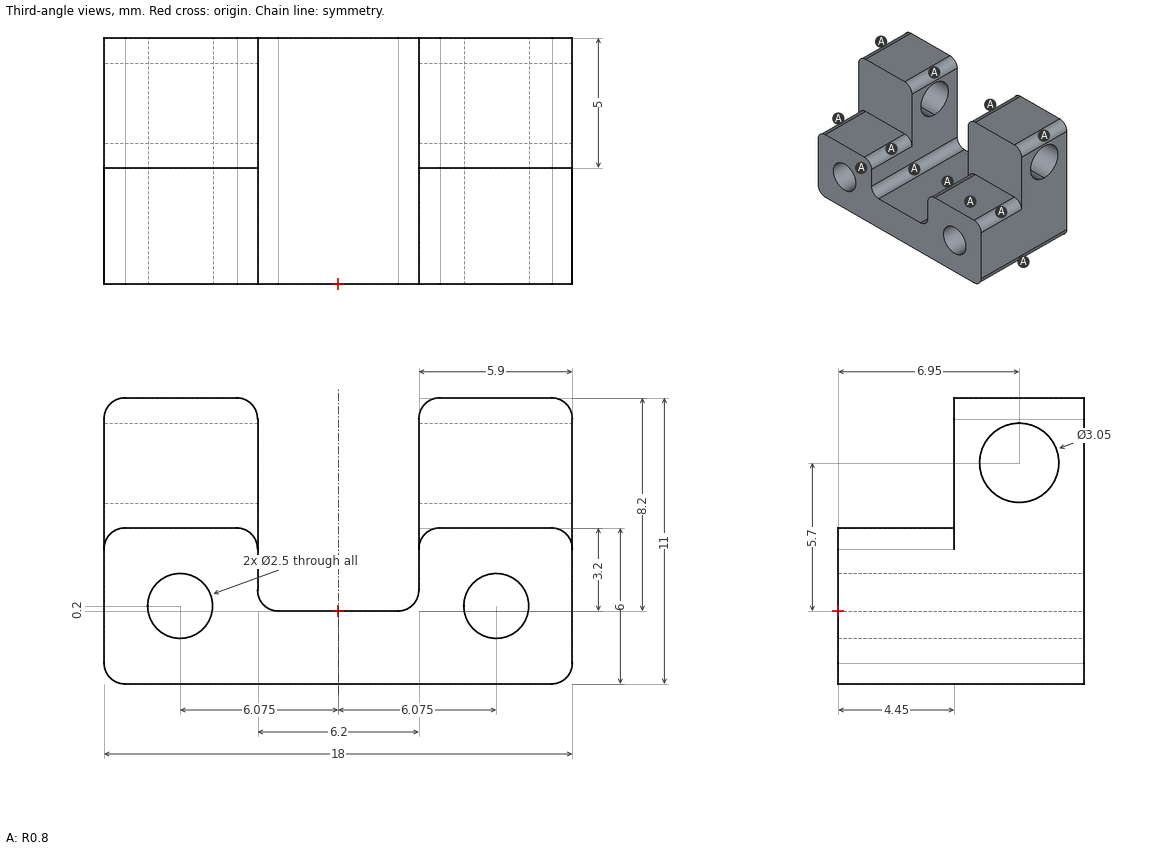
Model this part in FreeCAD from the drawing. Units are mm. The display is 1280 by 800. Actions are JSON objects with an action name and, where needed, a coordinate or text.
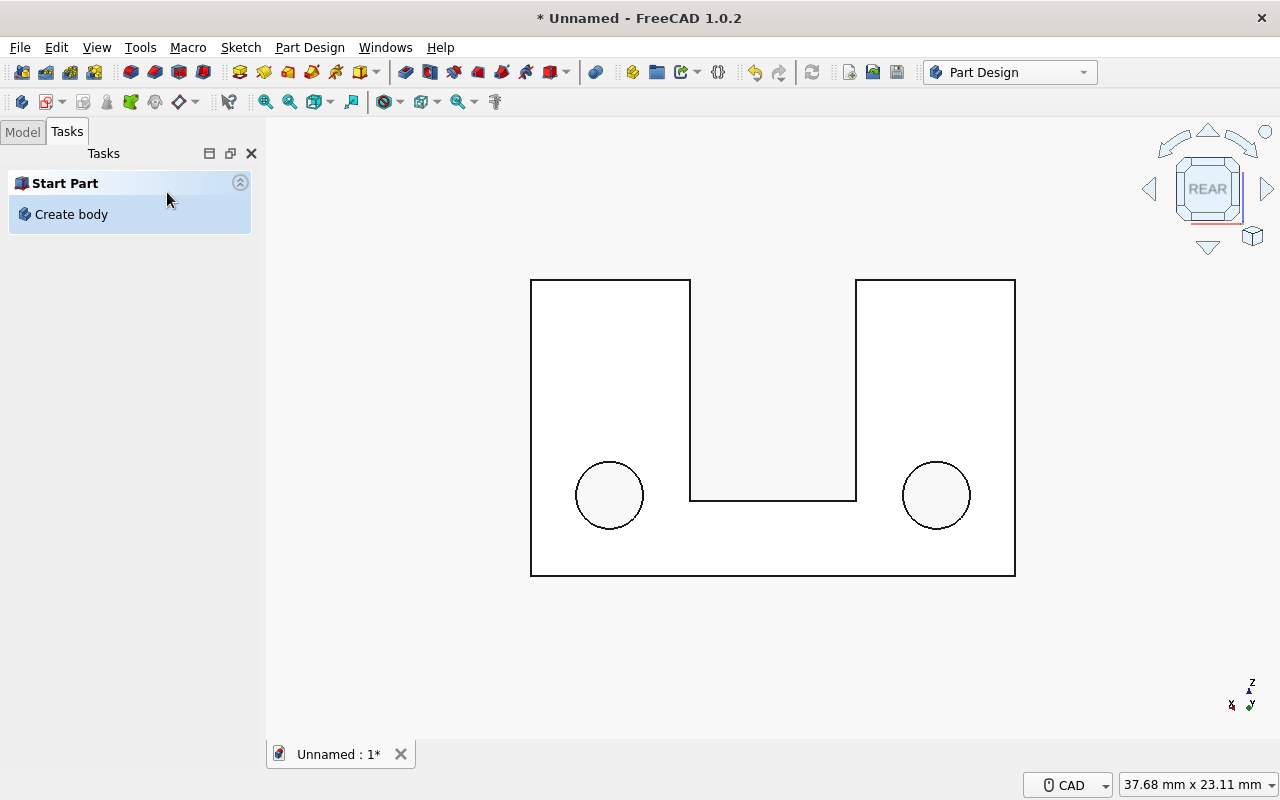
{"action": "key", "text": "6"}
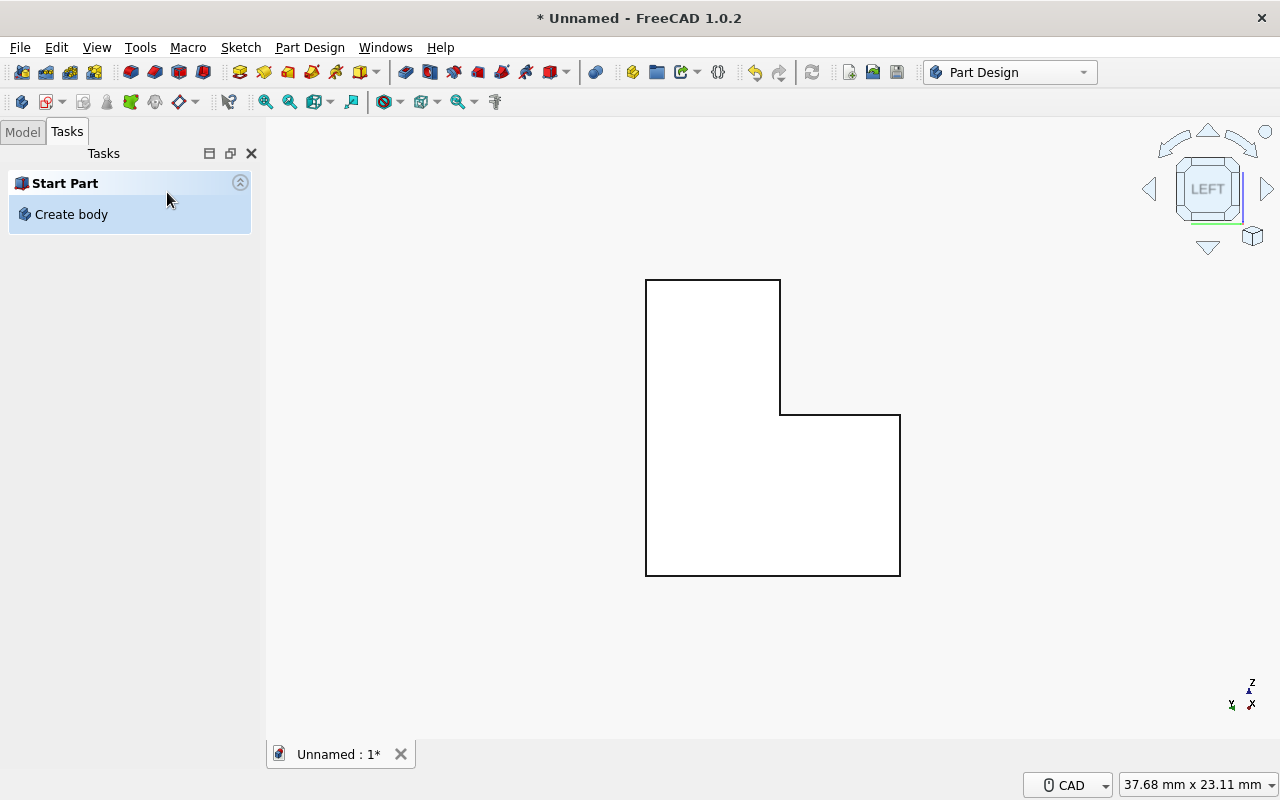
{"action": "left_click", "coordinate": [737, 469]}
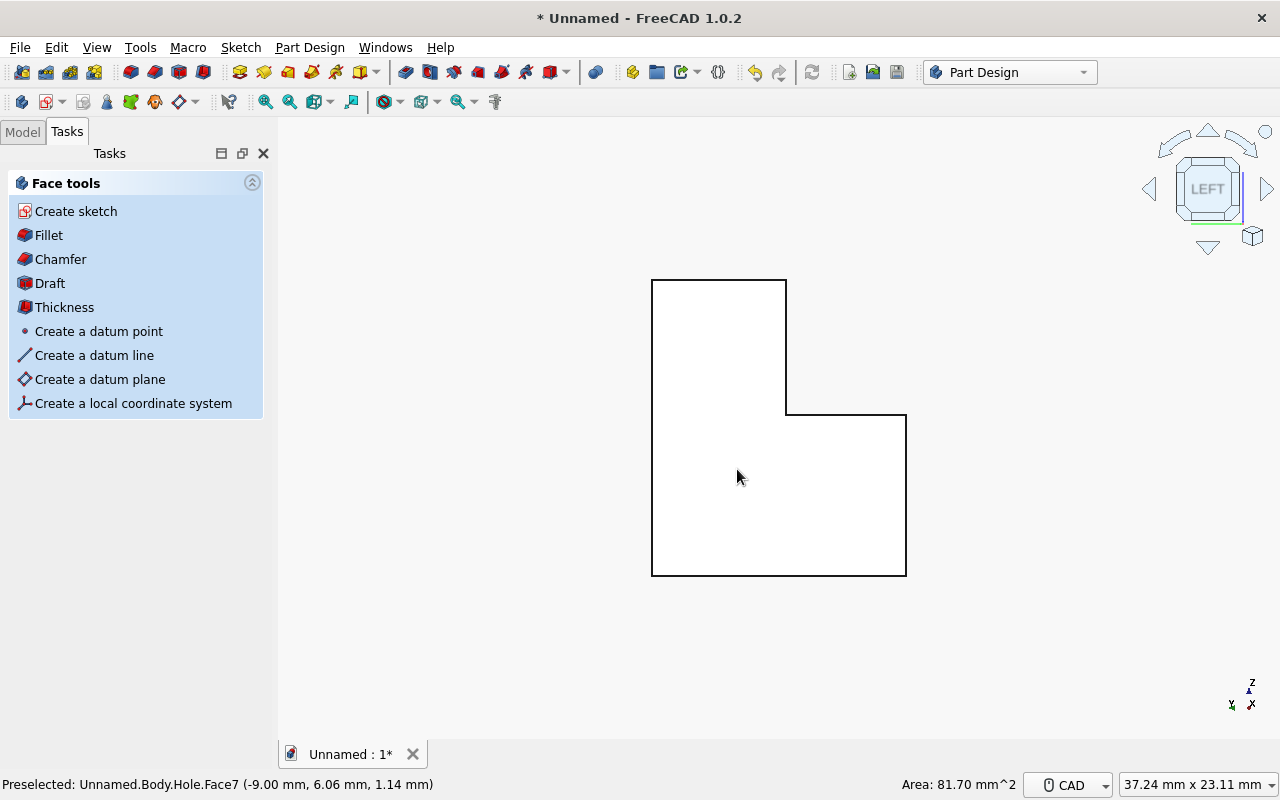
{"action": "left_click", "coordinate": [46, 102]}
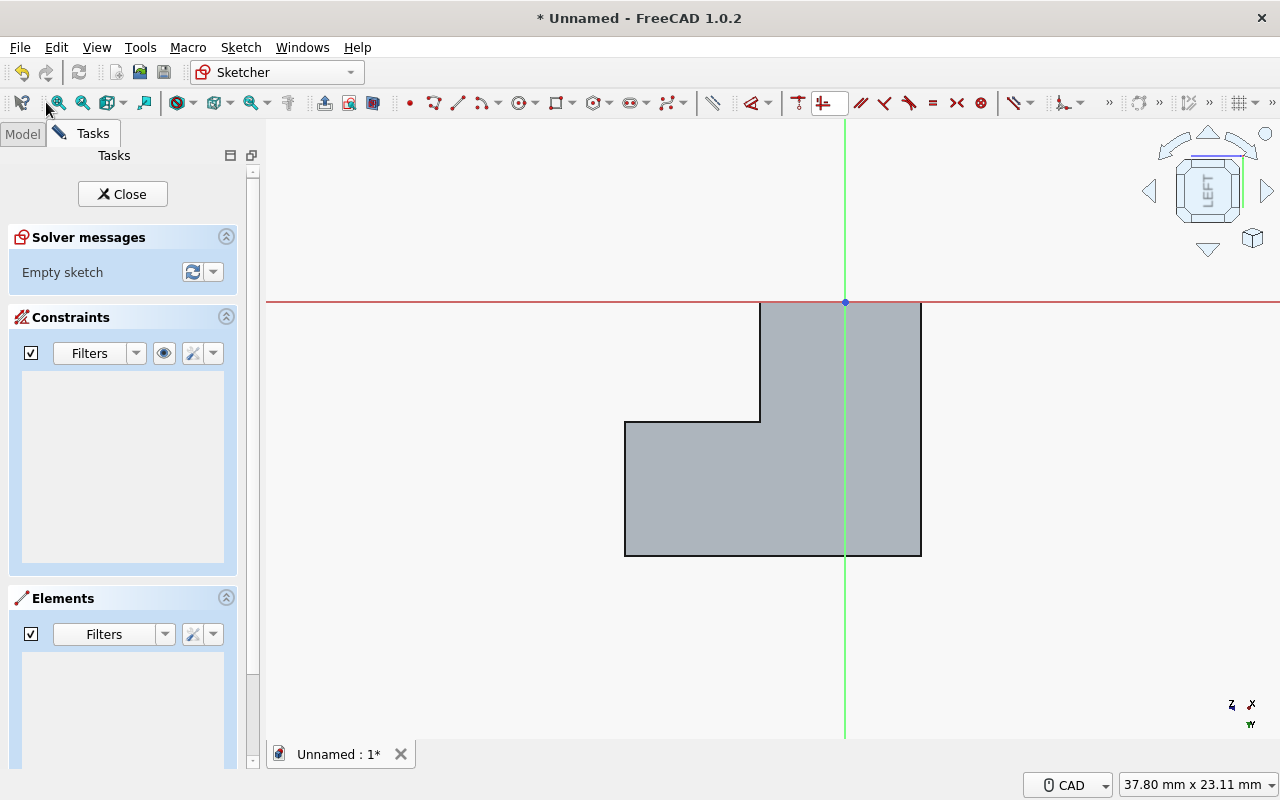
{"action": "scroll", "coordinate": [690, 504], "scroll_direction": "up", "scroll_amount": 8}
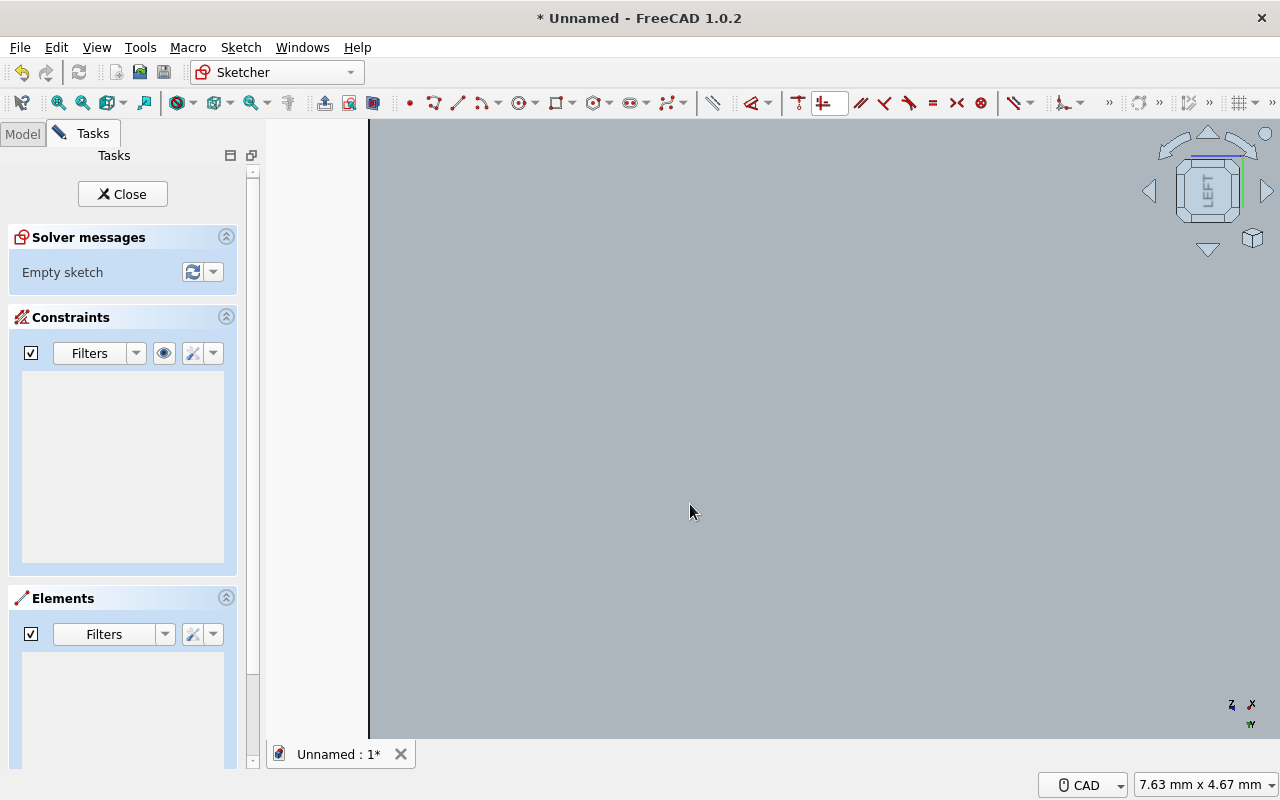
{"action": "left_click", "coordinate": [520, 104]}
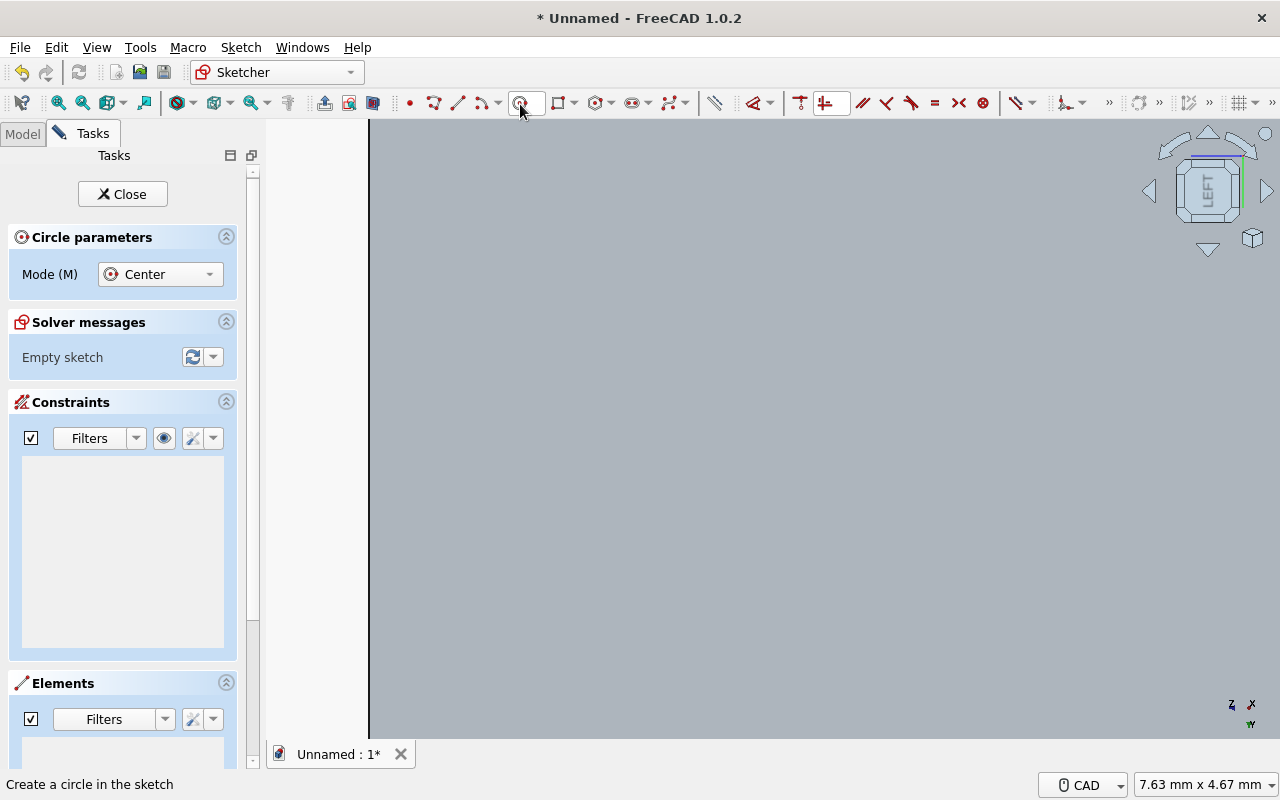
{"action": "left_click", "coordinate": [701, 426]}
{"action": "mouse_move", "coordinate": [844, 282]}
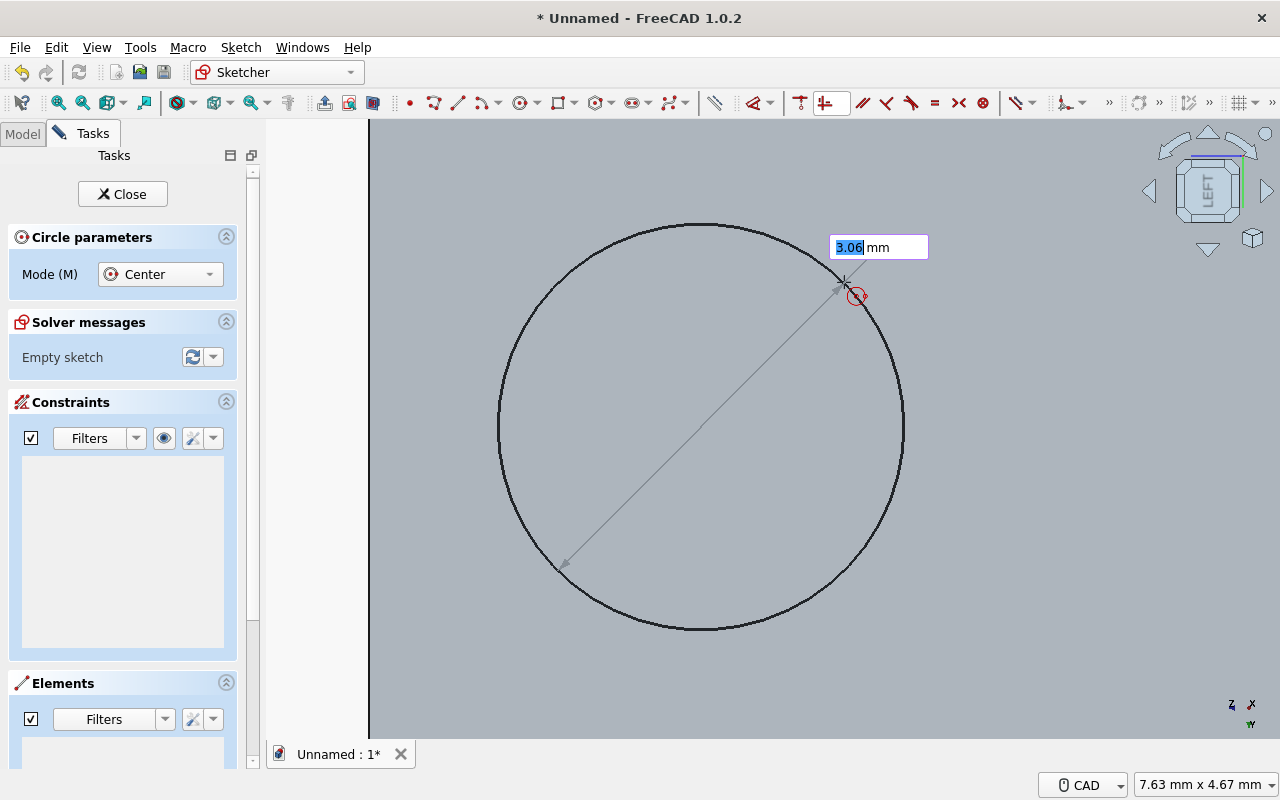
{"action": "type", "text": "3.05"}
{"action": "key", "text": "Return"}
{"action": "key", "text": "Escape"}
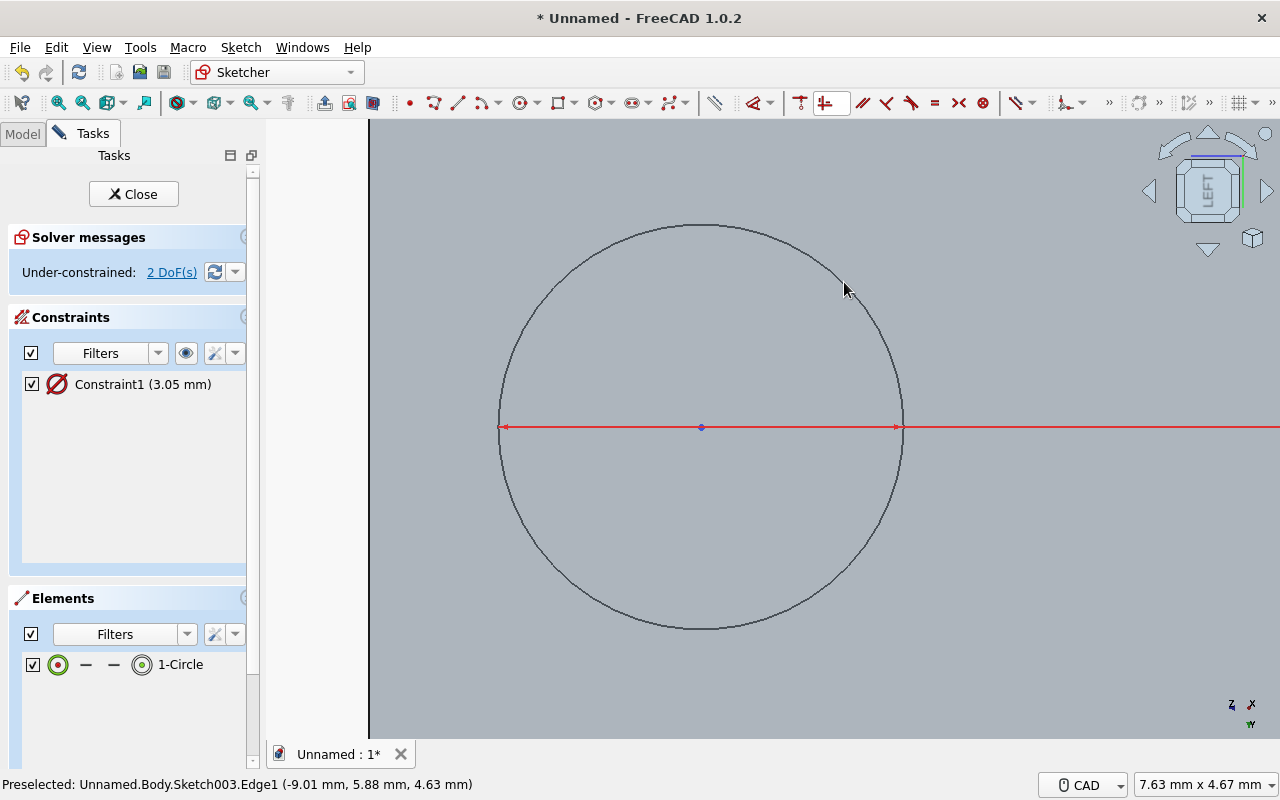
{"action": "left_click", "coordinate": [754, 104]}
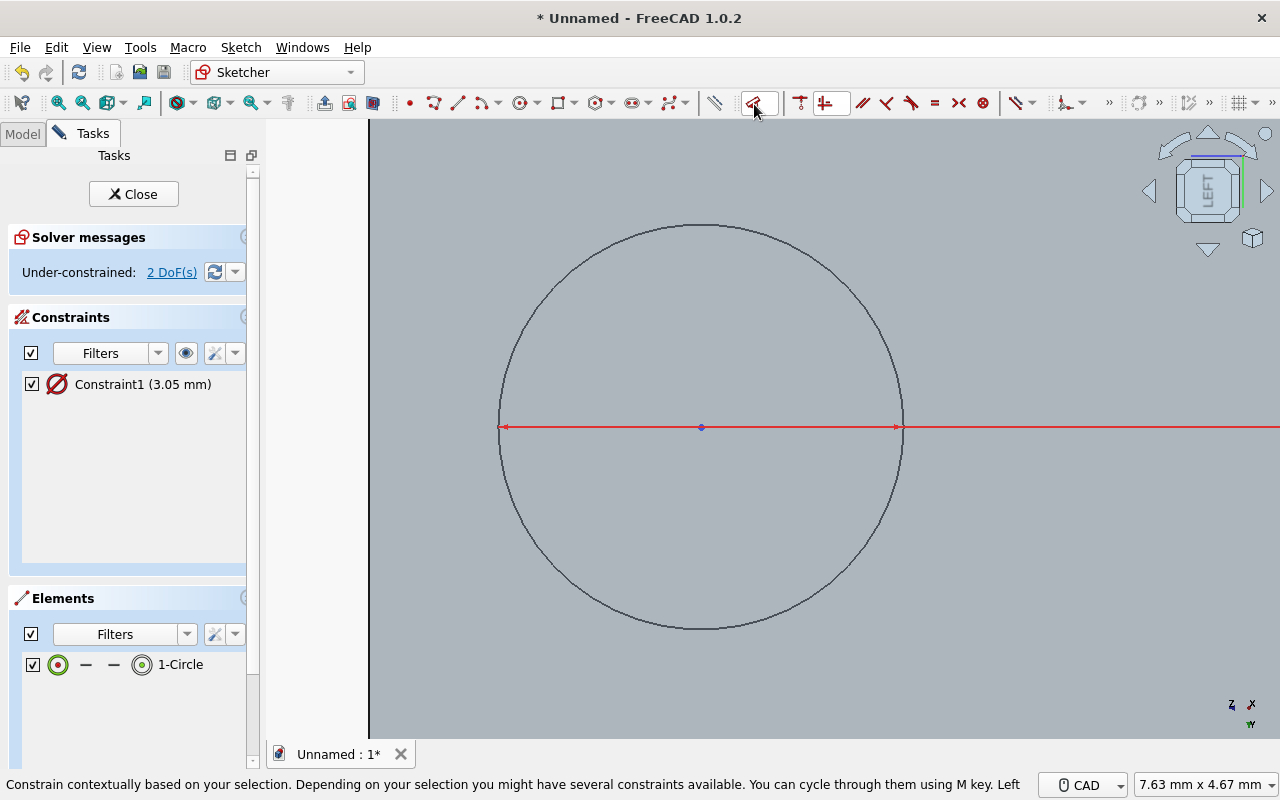
{"action": "left_click", "coordinate": [701, 427]}
{"action": "left_click", "coordinate": [813, 461]}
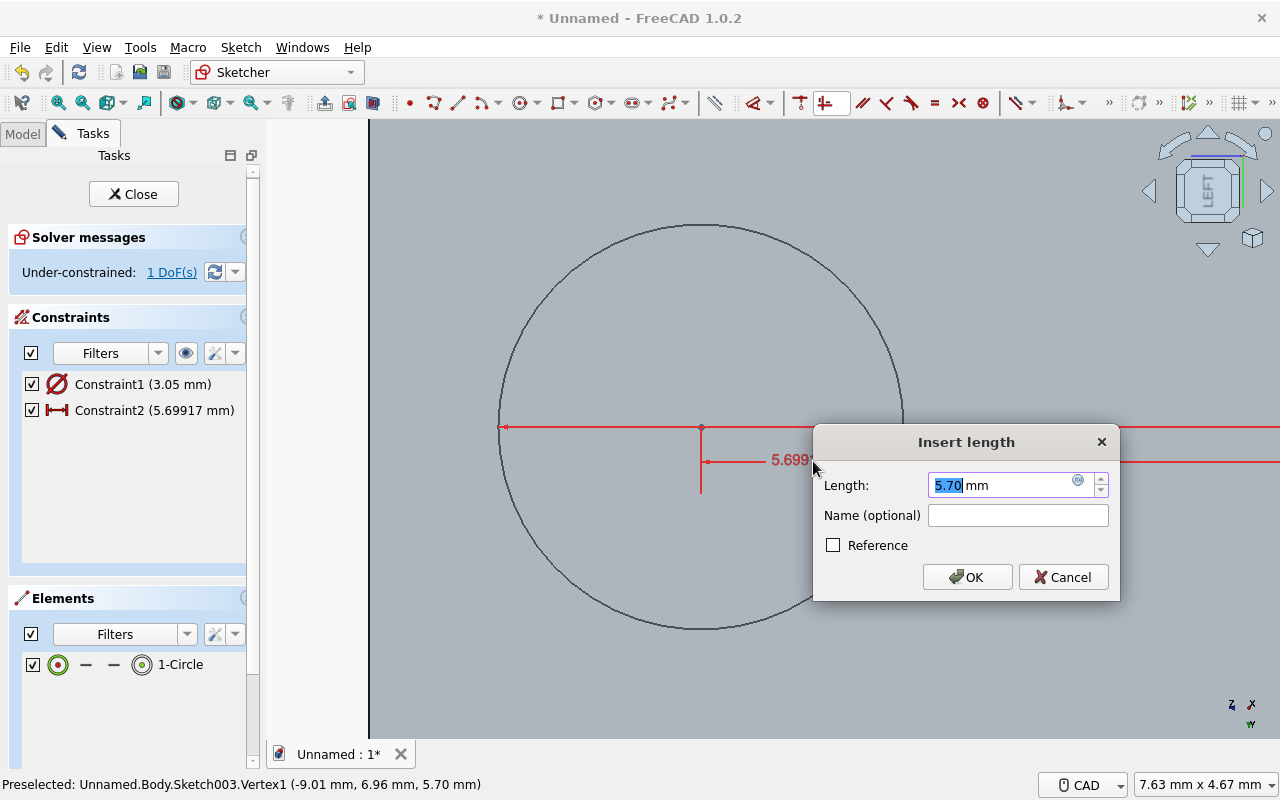
{"action": "type", "text": "5.7"}
{"action": "key", "text": "Return"}